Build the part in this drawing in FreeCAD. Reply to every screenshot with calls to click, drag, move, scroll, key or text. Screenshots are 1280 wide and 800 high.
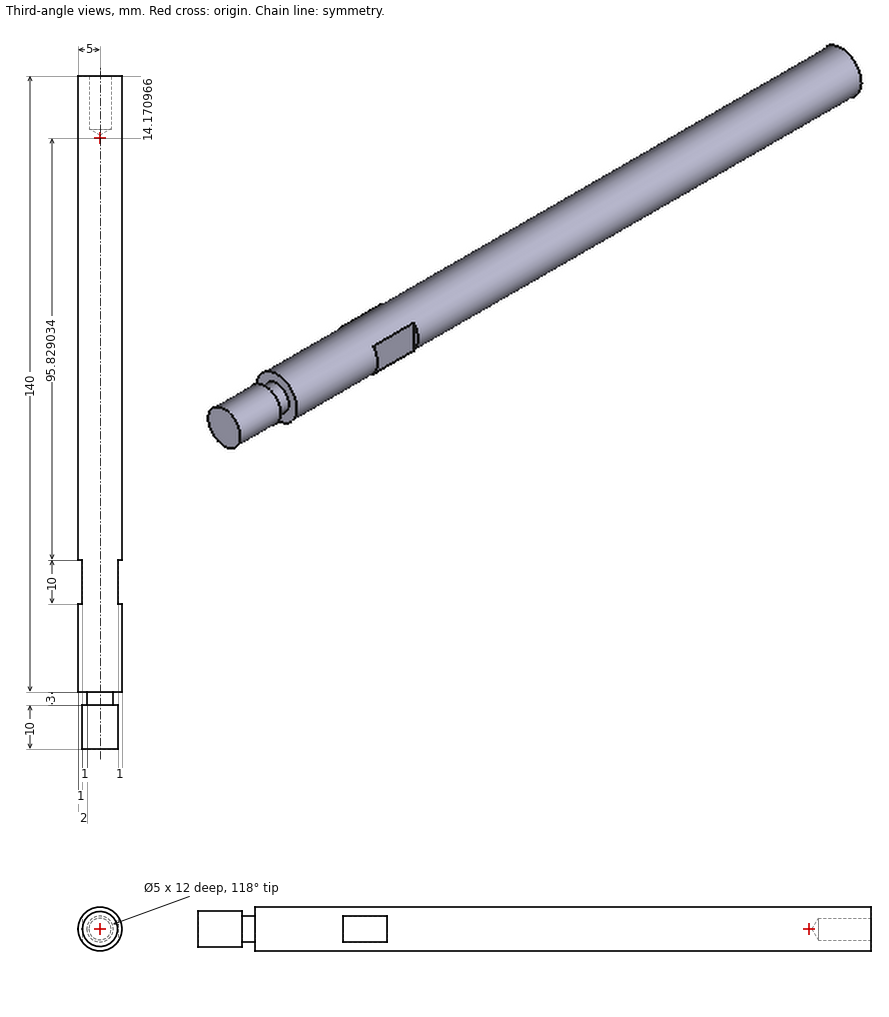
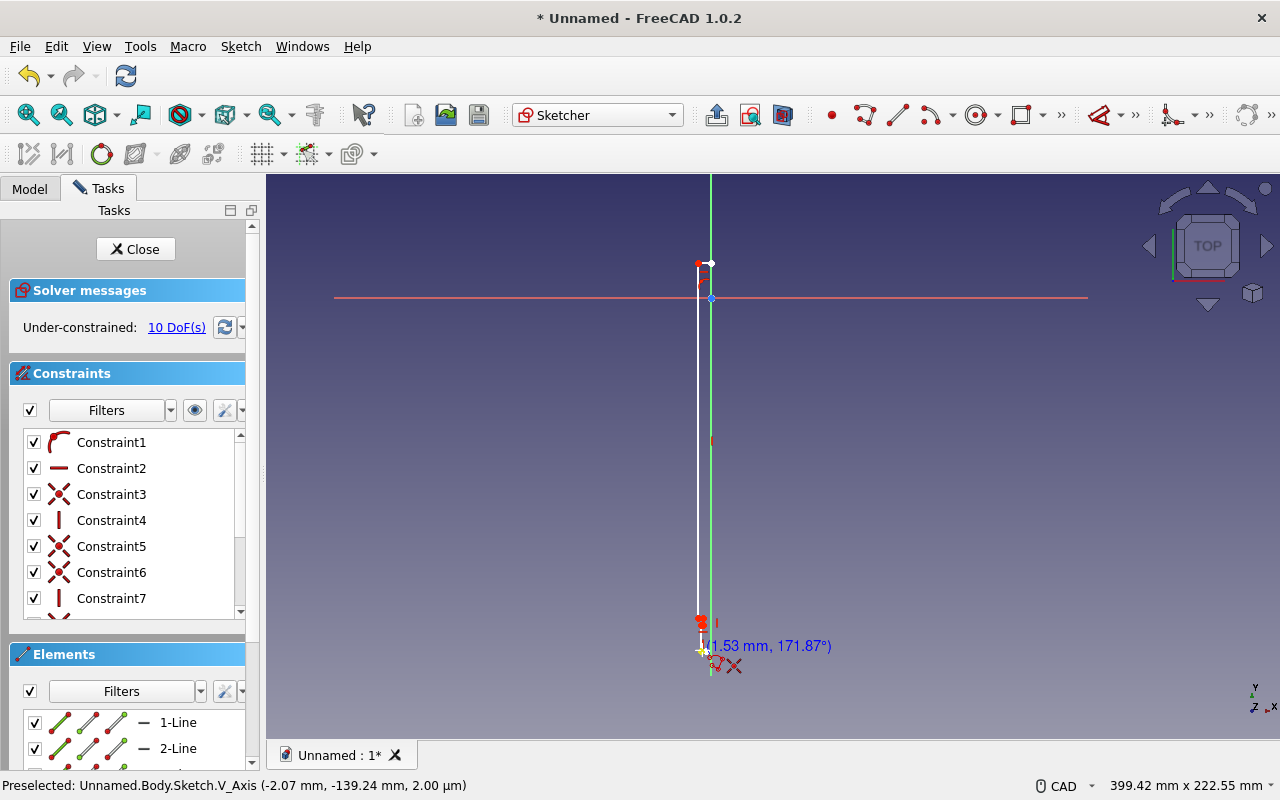
scroll(711, 263, up, 5)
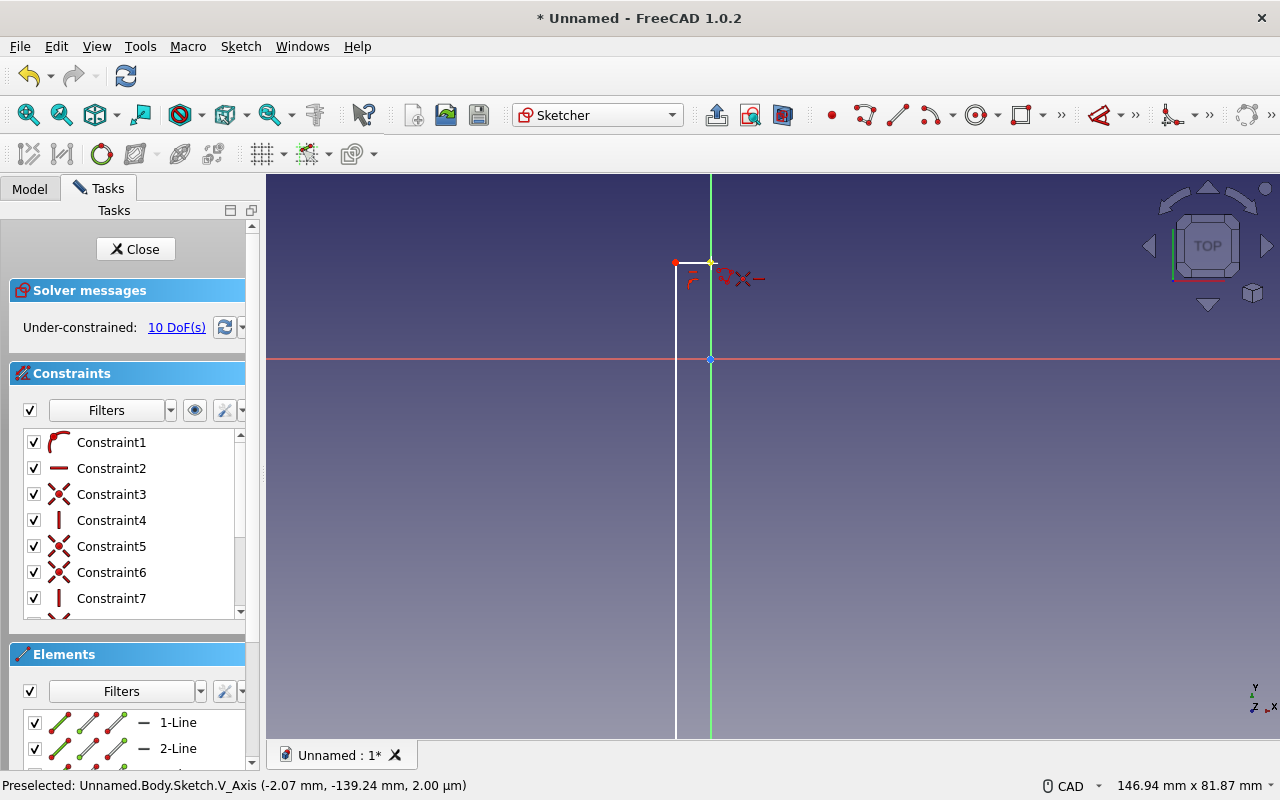
click(711, 263)
key(Escape)
key(Escape)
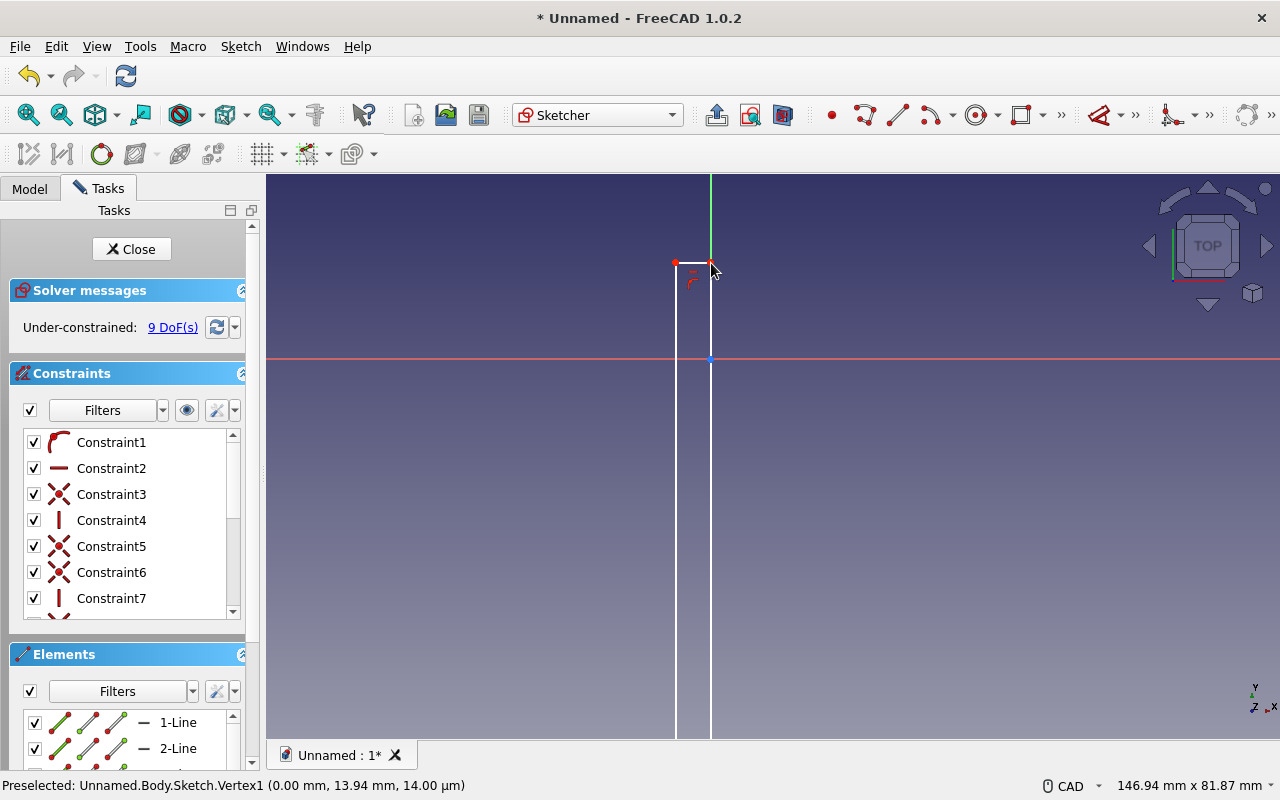
scroll(711, 263, down, 5)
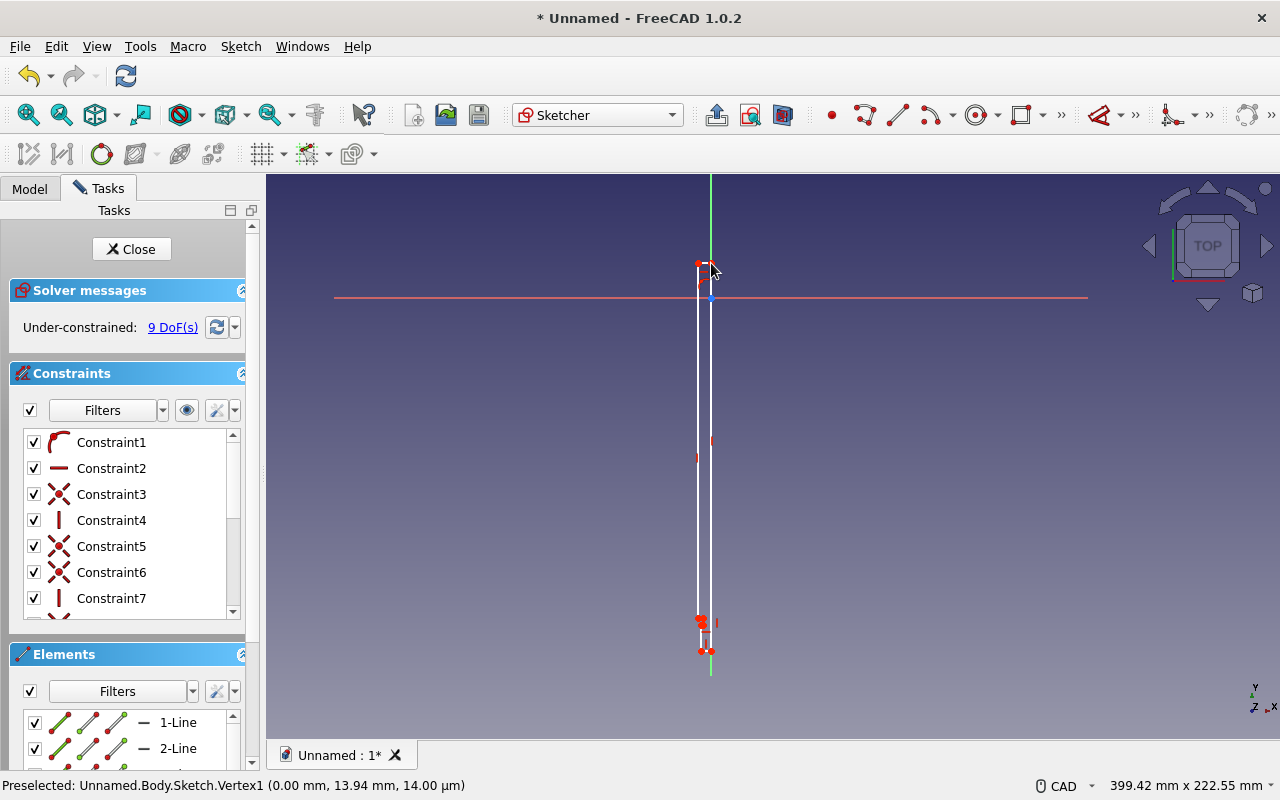
scroll(701, 618, up, 9)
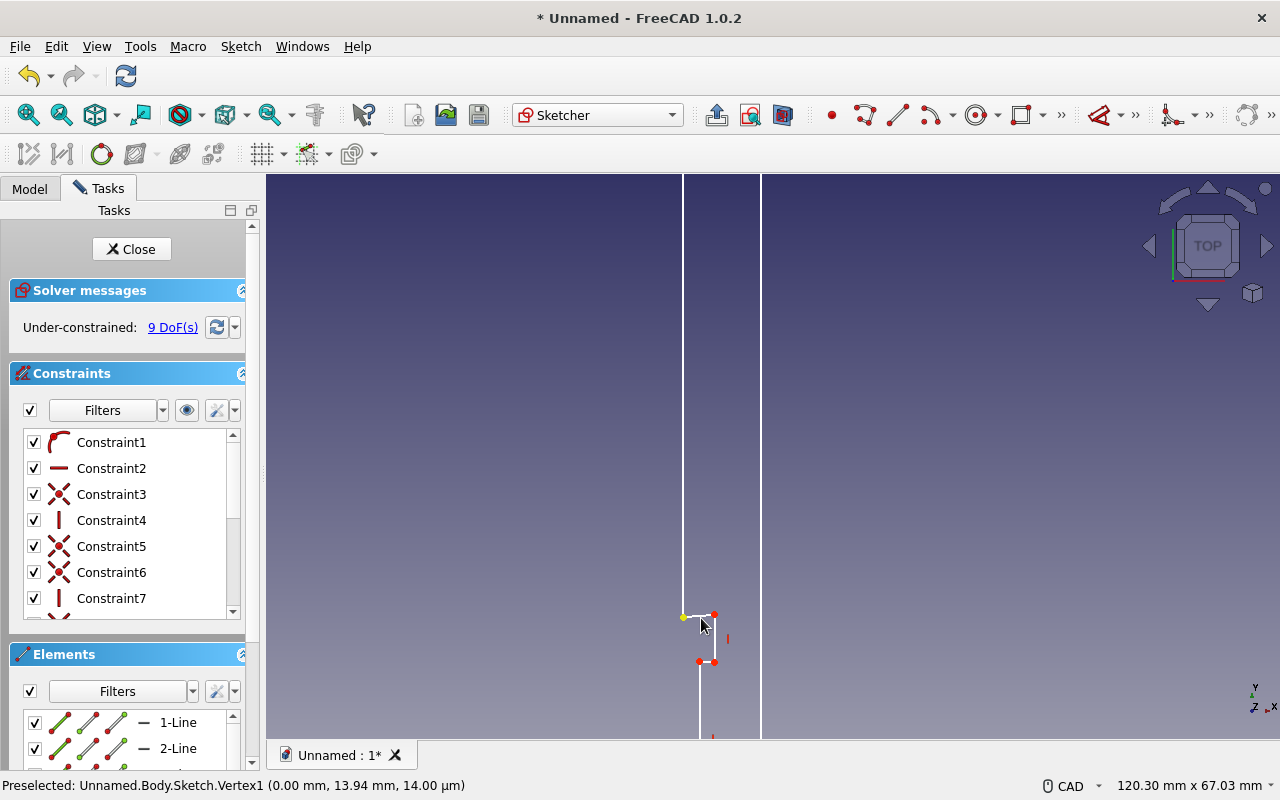
click(699, 616)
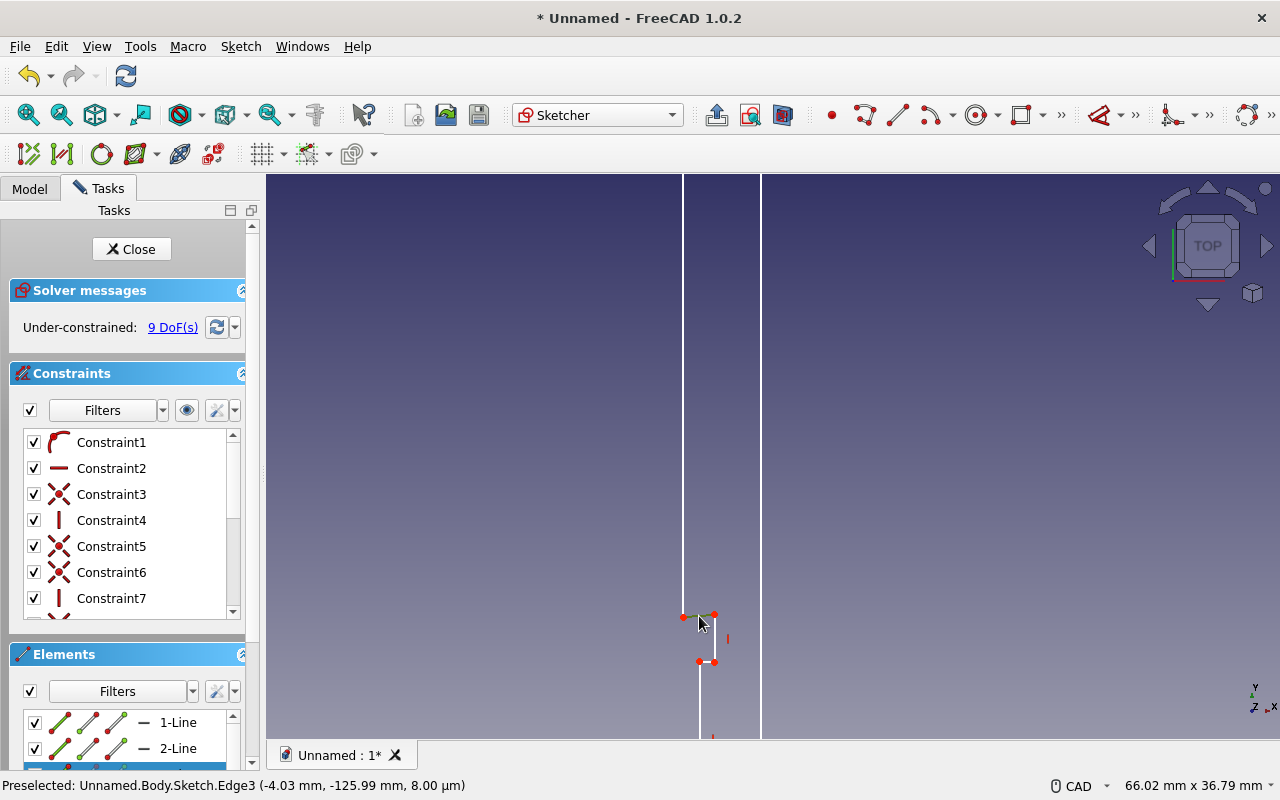
key(h)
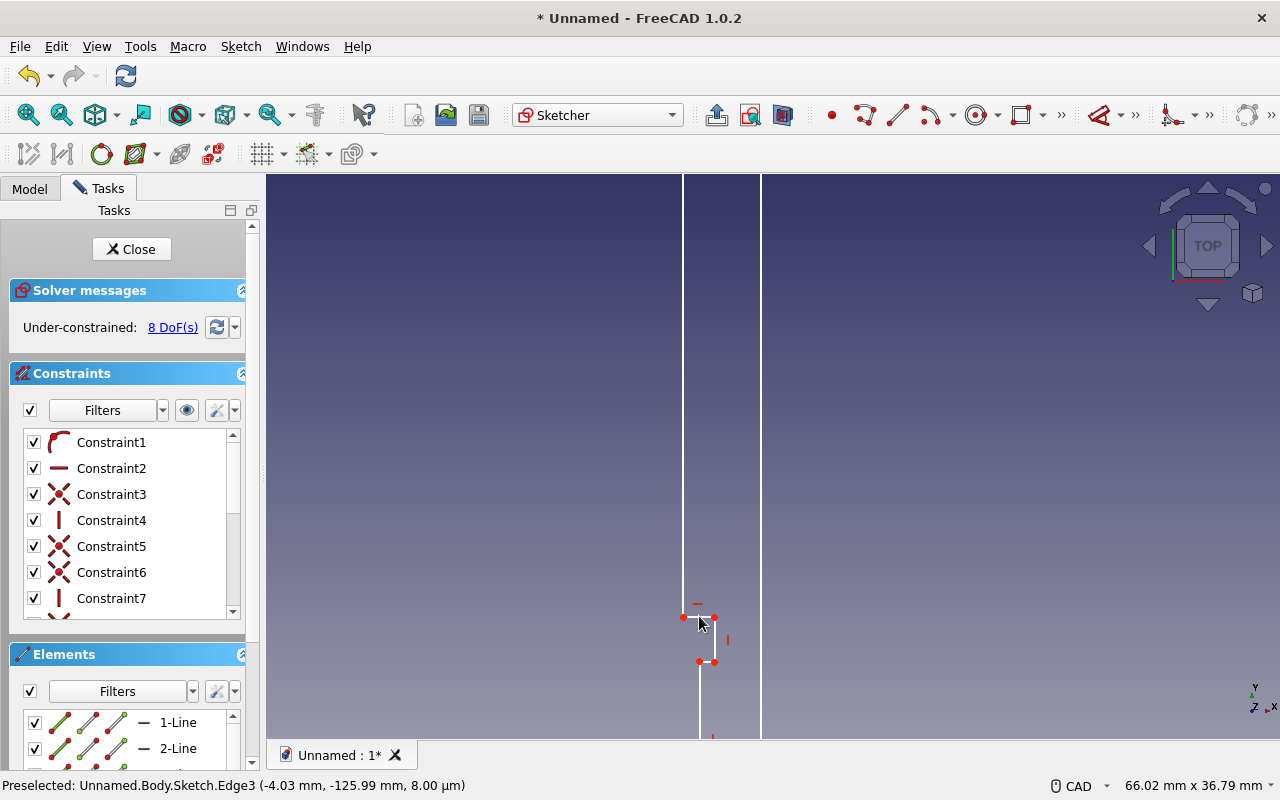
scroll(707, 662, up, 4)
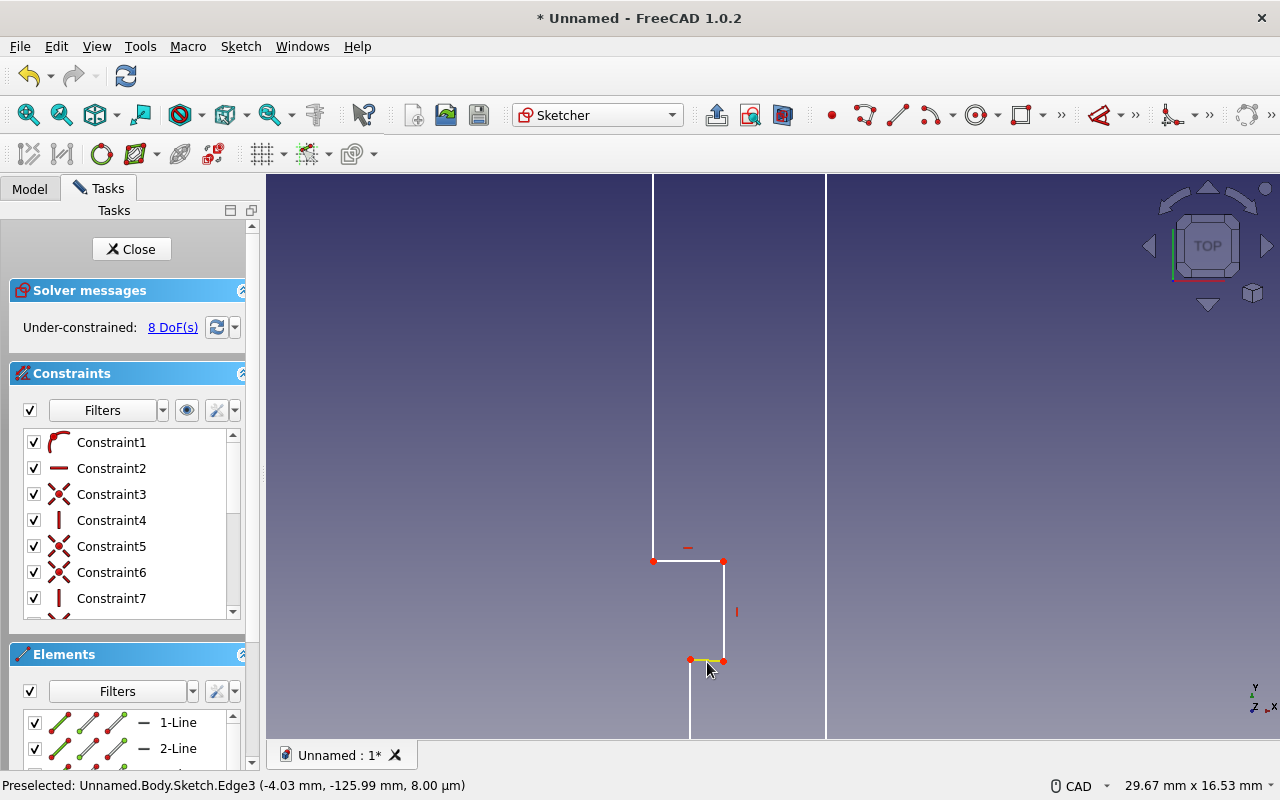
click(707, 660)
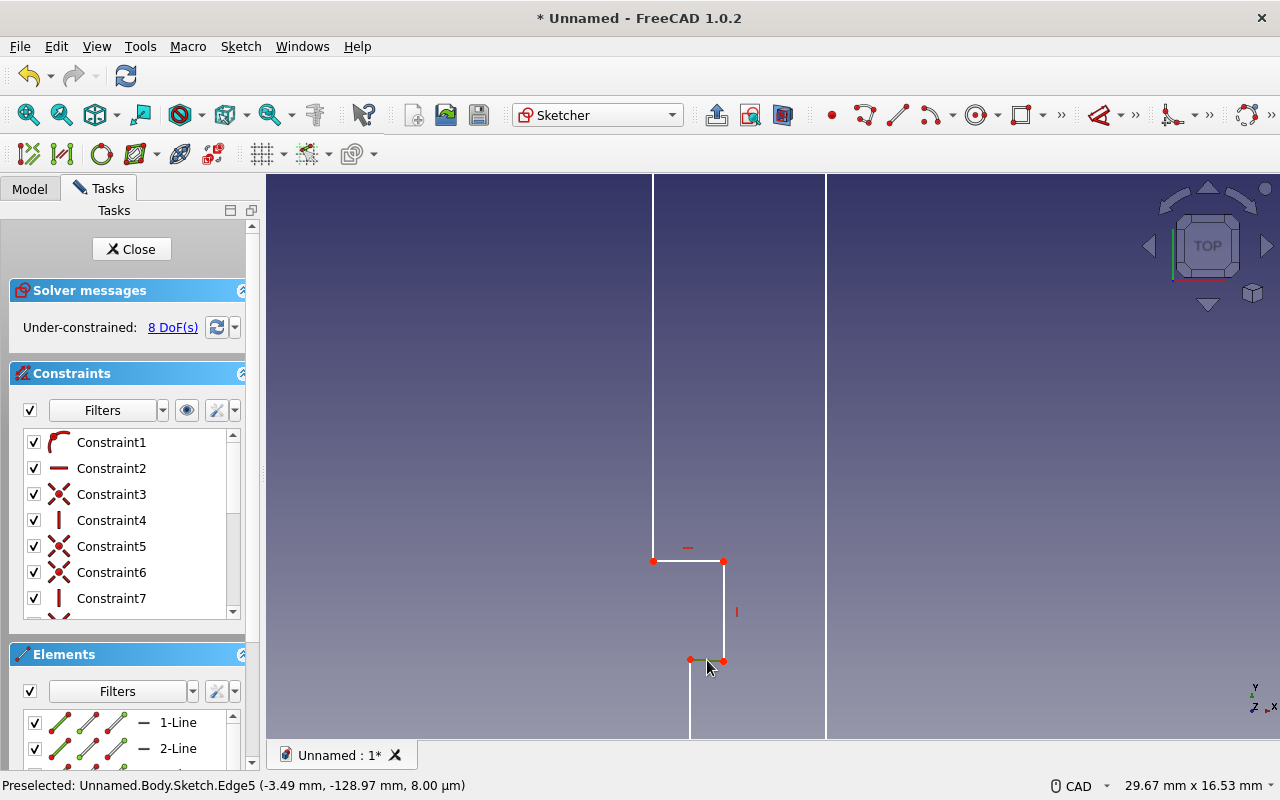
key(h)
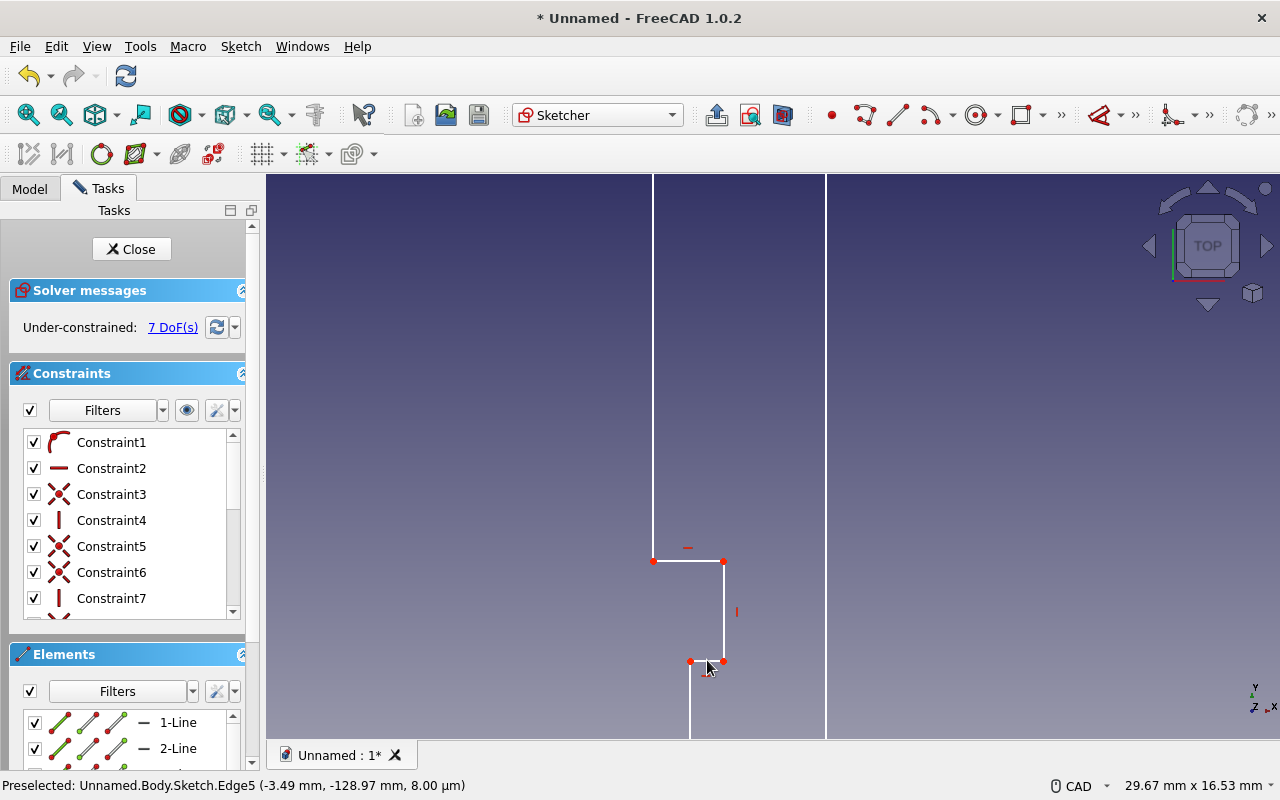
scroll(702, 623, down, 13)